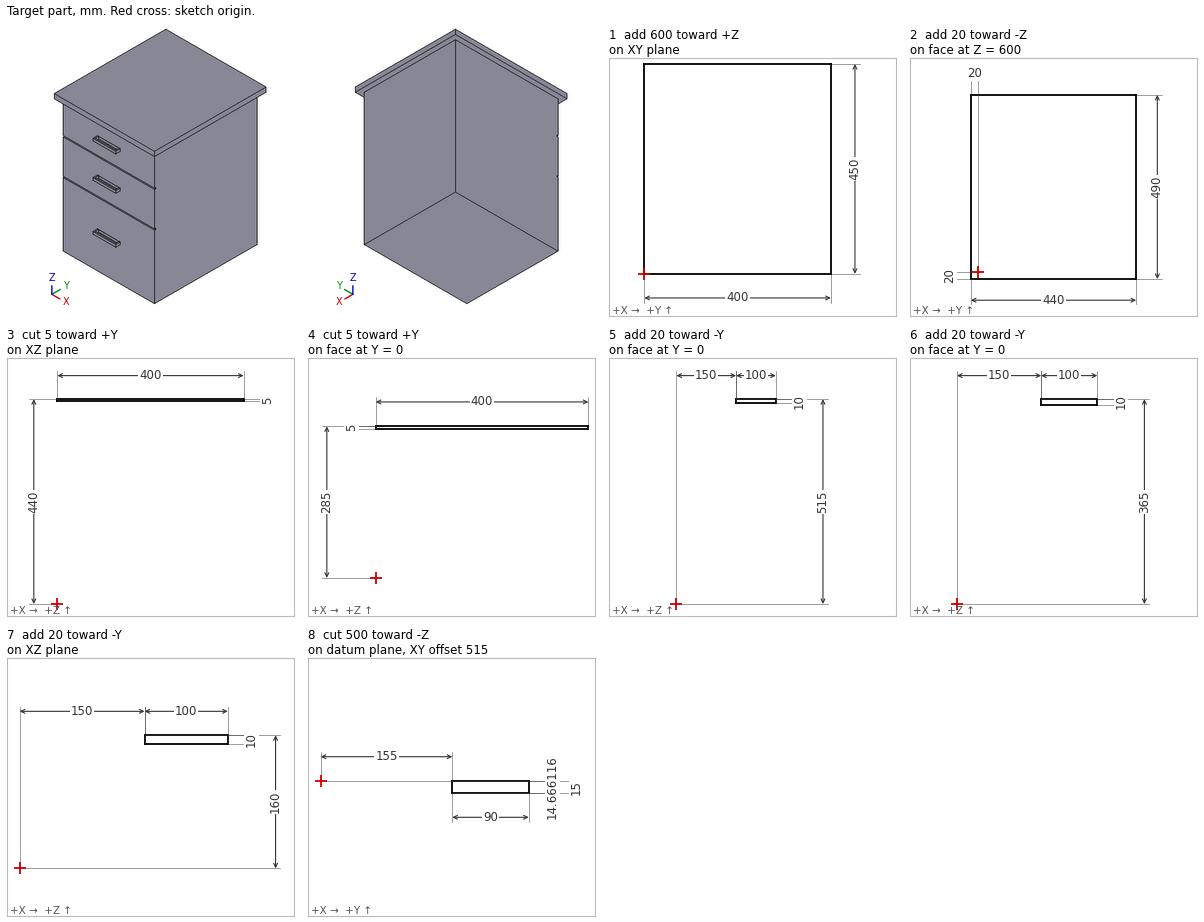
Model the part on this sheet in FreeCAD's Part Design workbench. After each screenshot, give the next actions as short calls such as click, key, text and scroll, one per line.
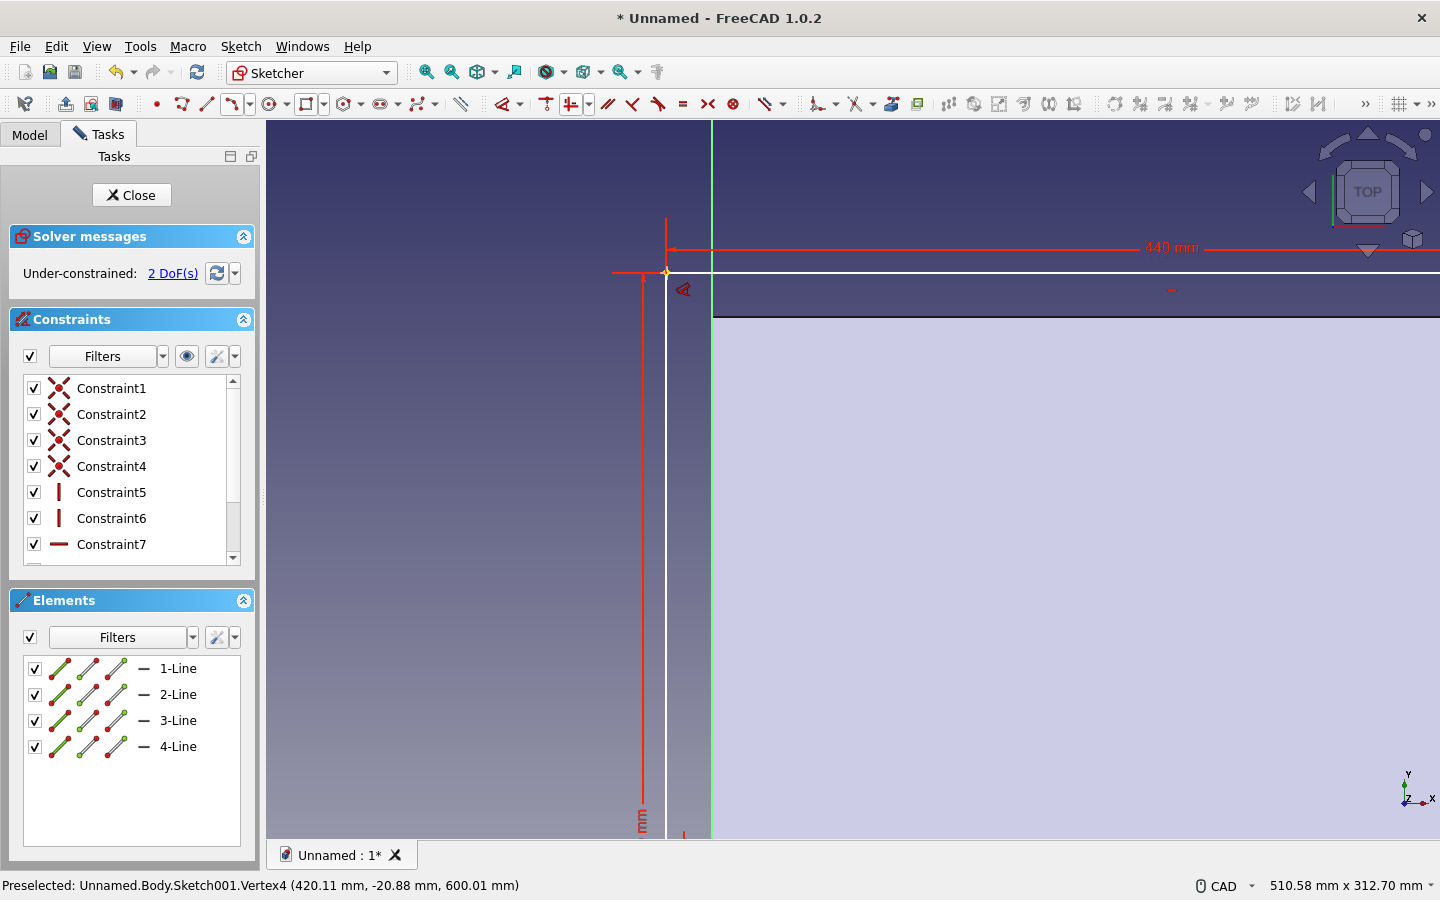
click(666, 273)
click(689, 239)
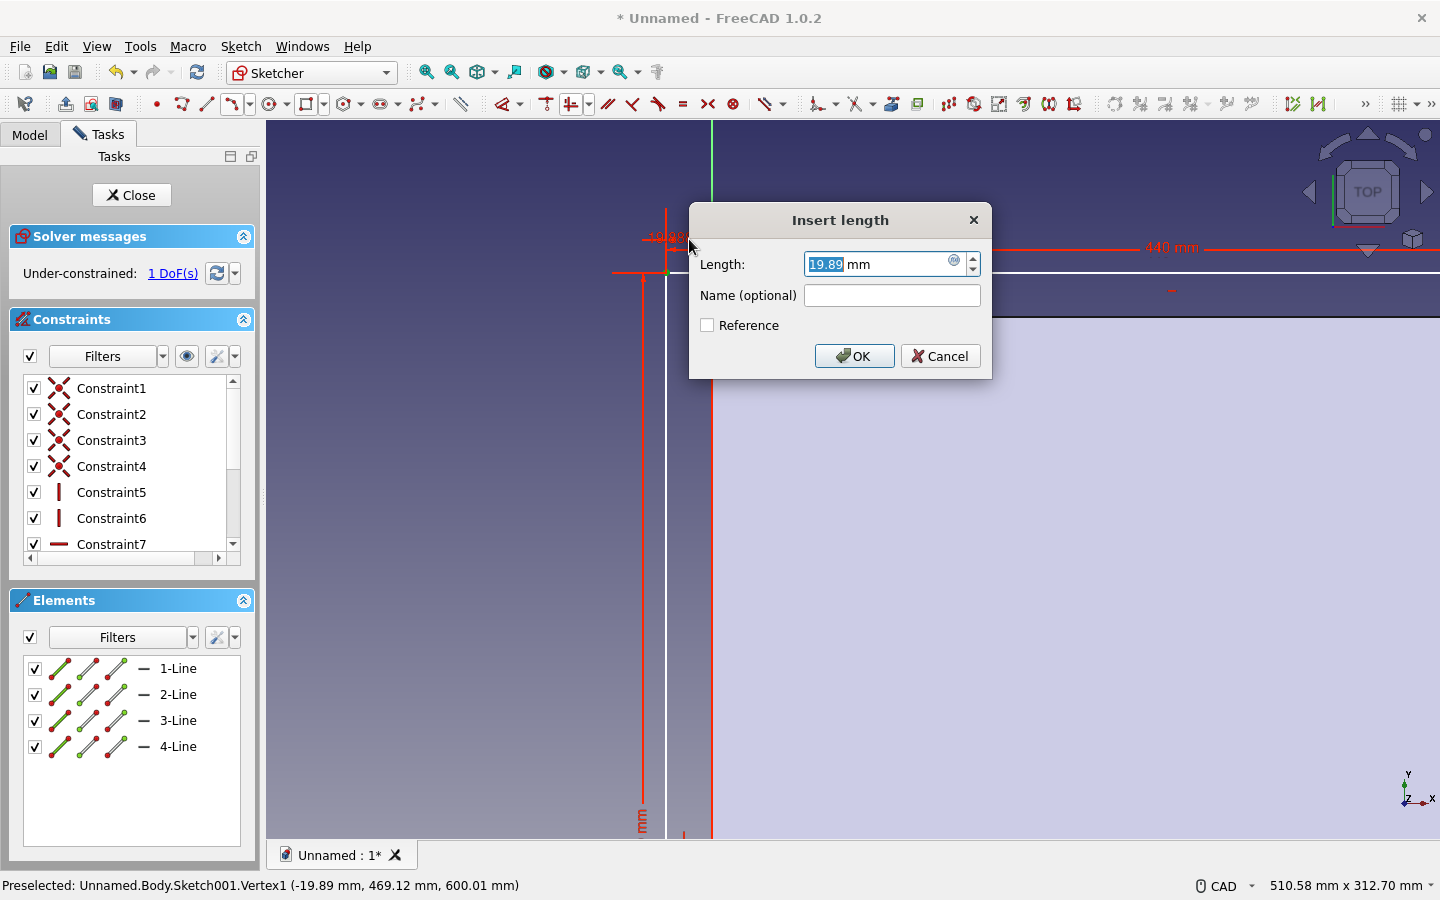
text(20)
key(Return)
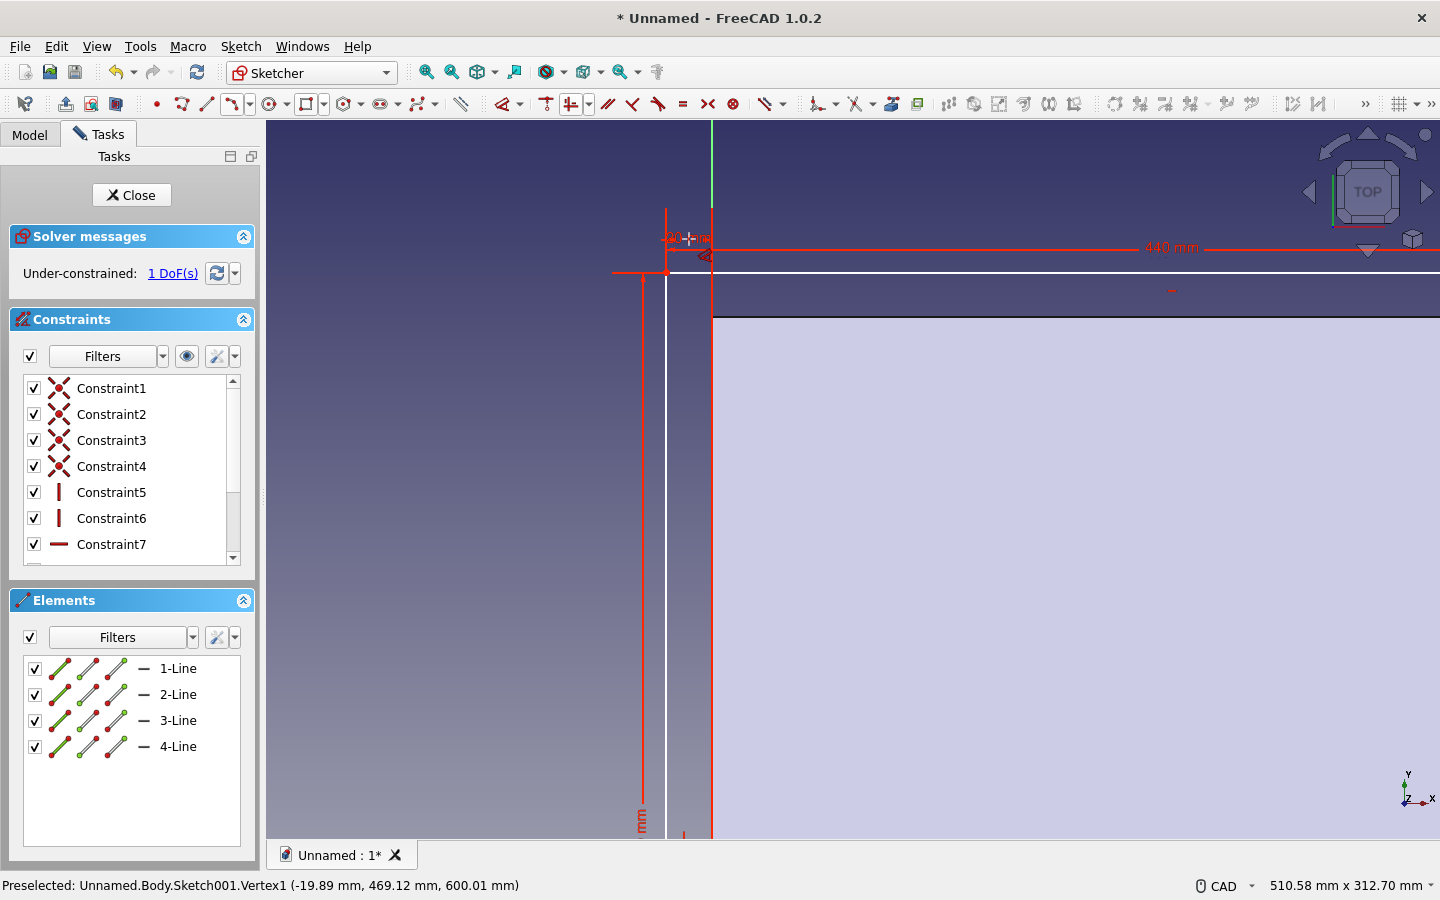
scroll(468, 190, down, 4)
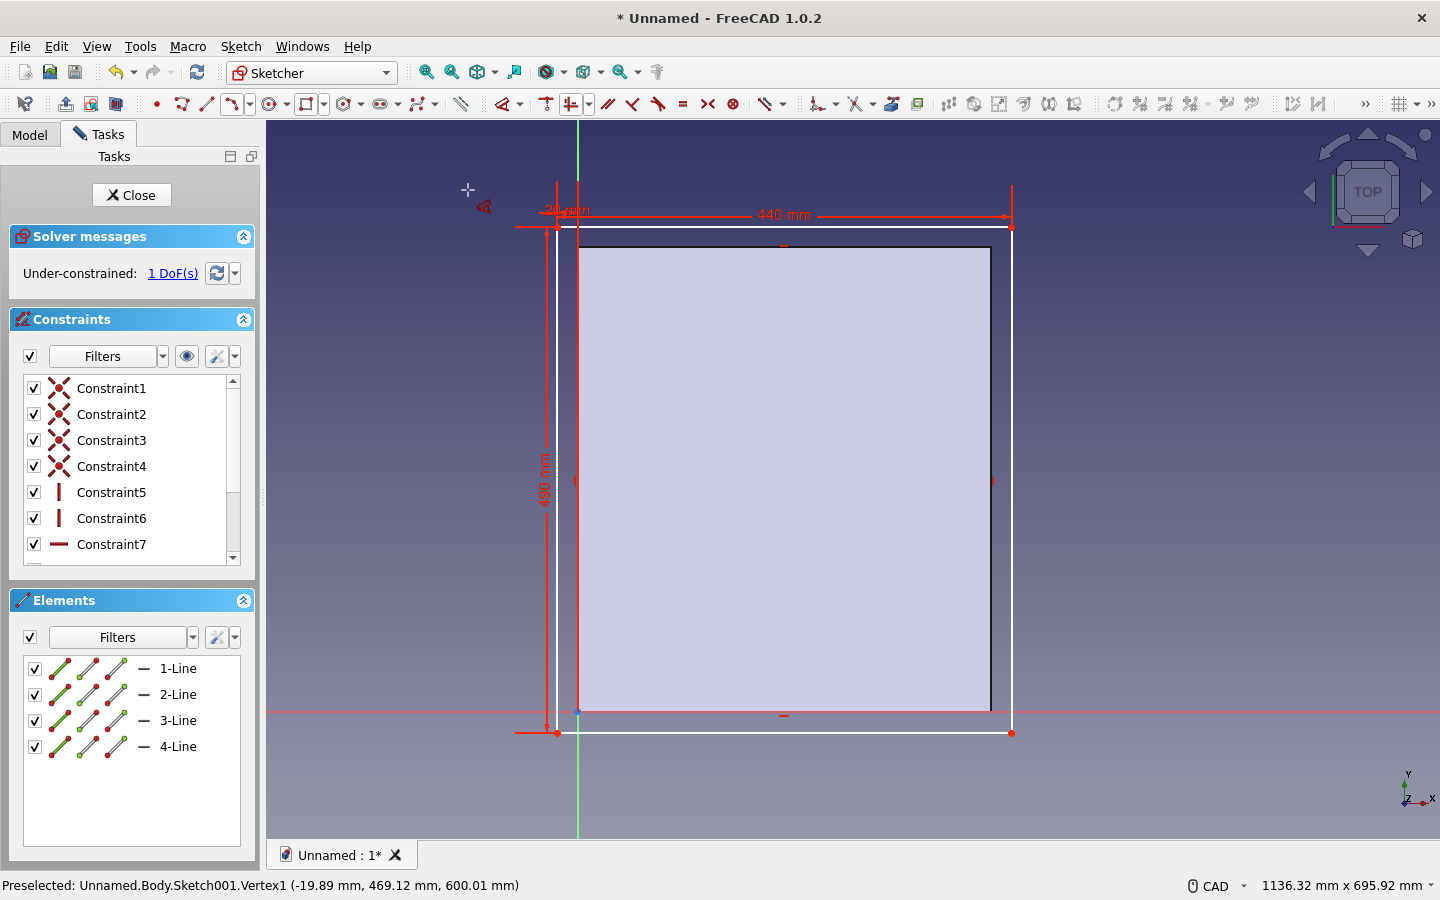
scroll(557, 733, up, 4)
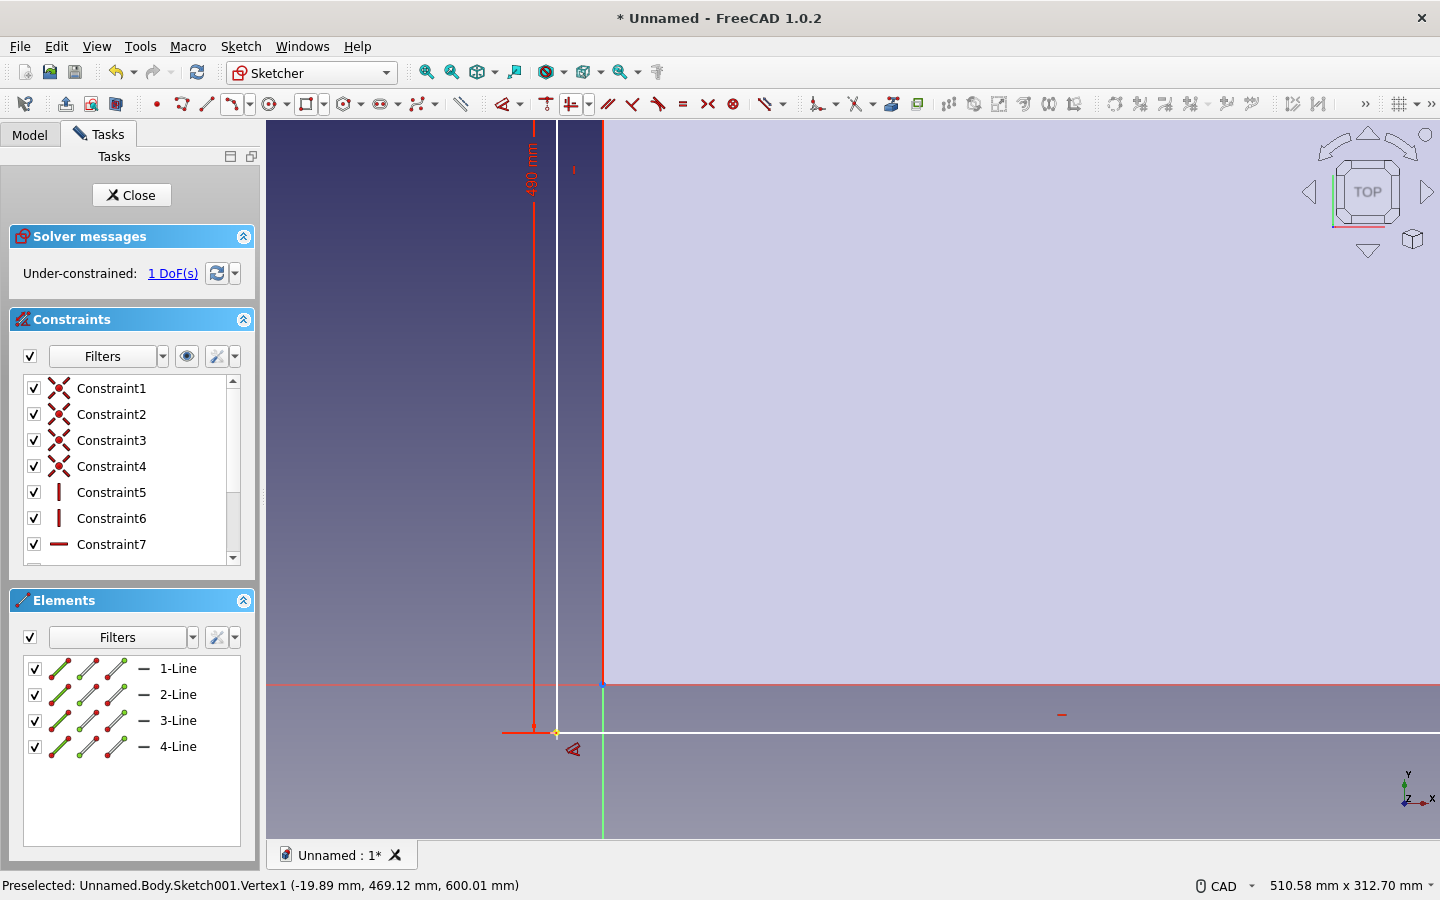
click(557, 733)
click(523, 709)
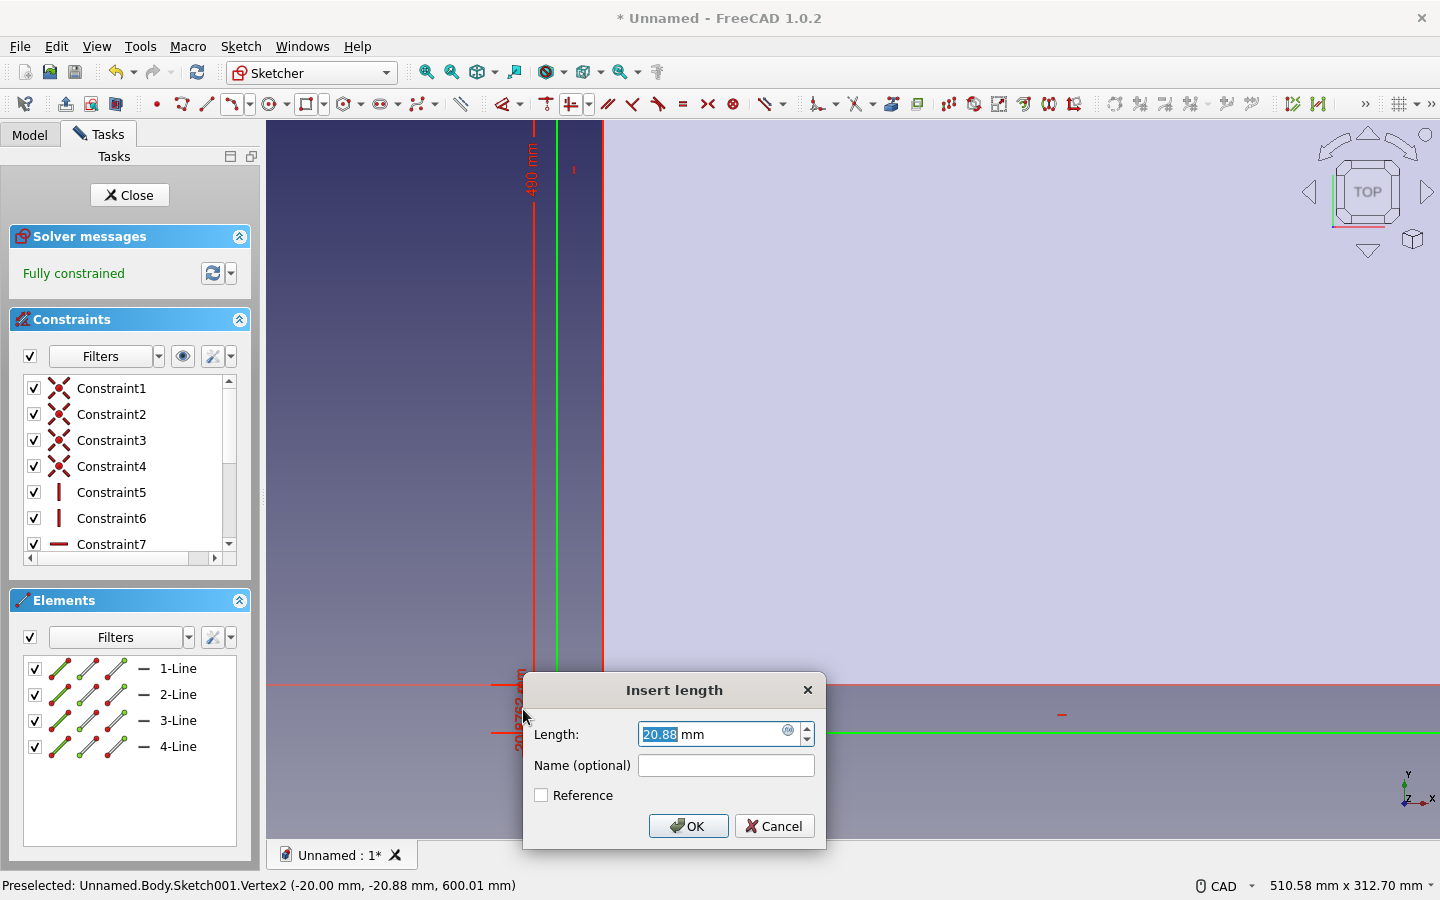
text(20)
key(Return)
key(Escape)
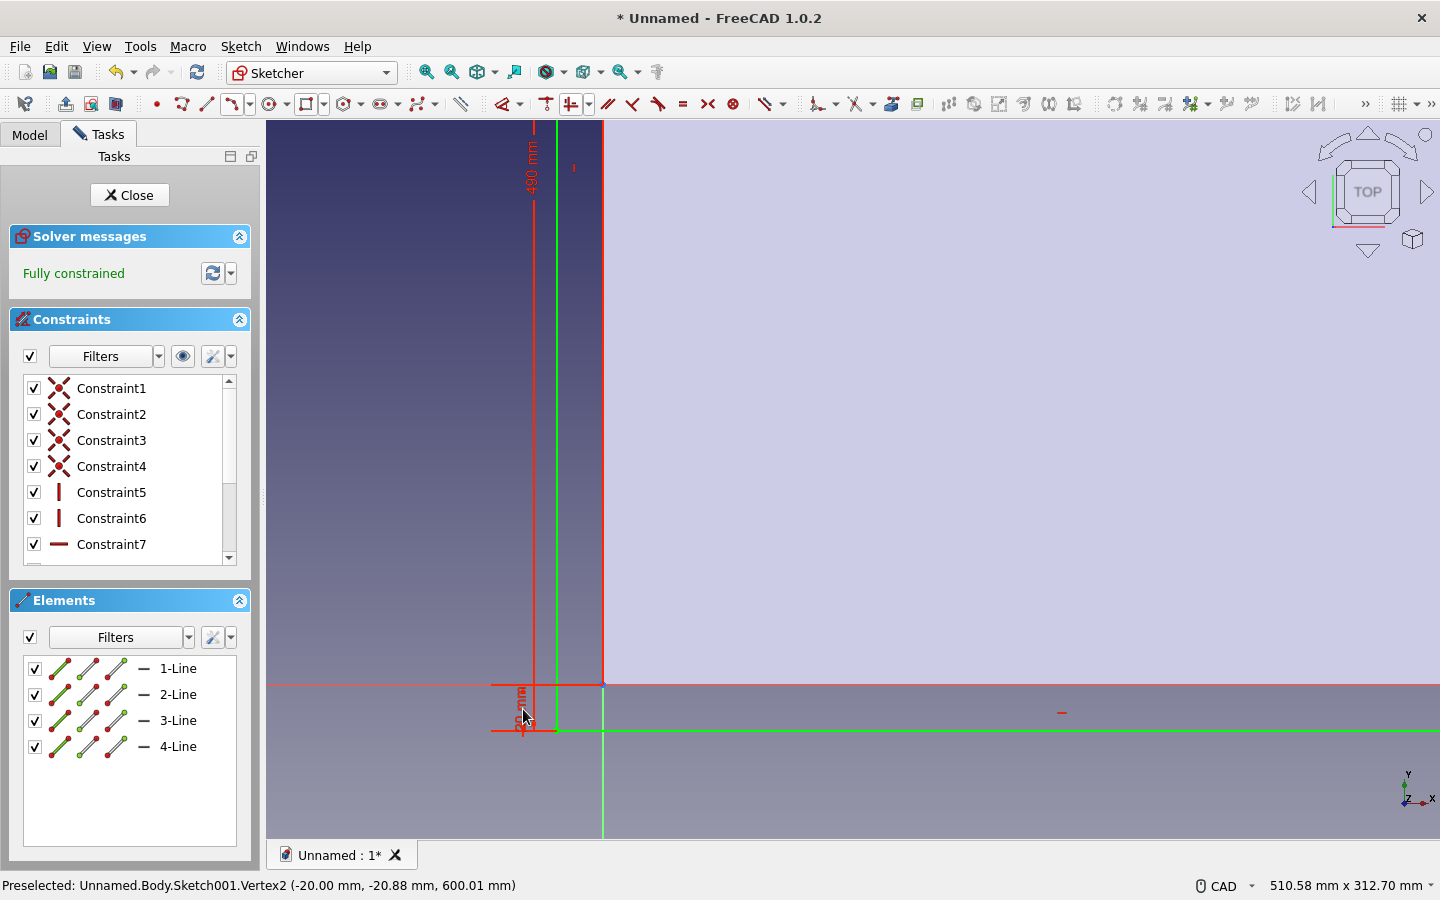
click(130, 195)